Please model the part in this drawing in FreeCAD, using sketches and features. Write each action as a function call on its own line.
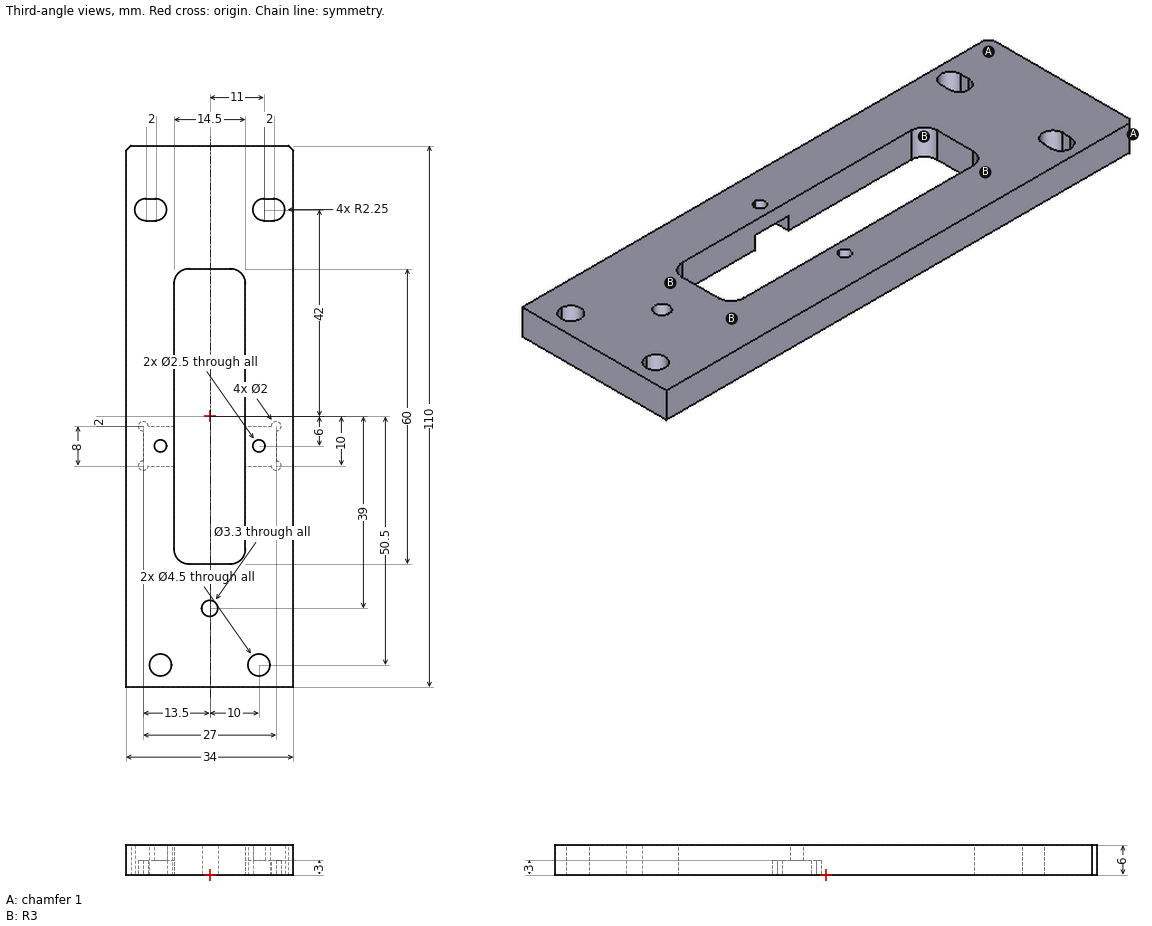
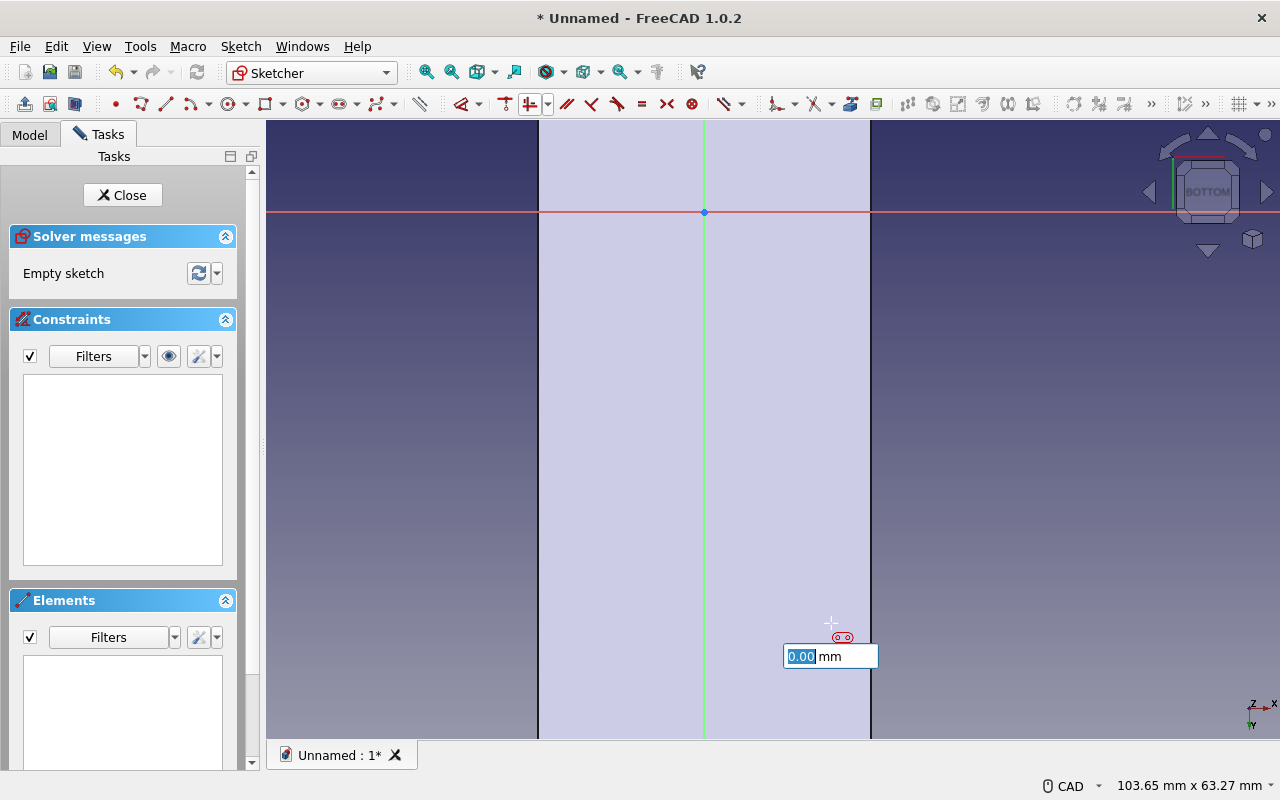
click(822, 645)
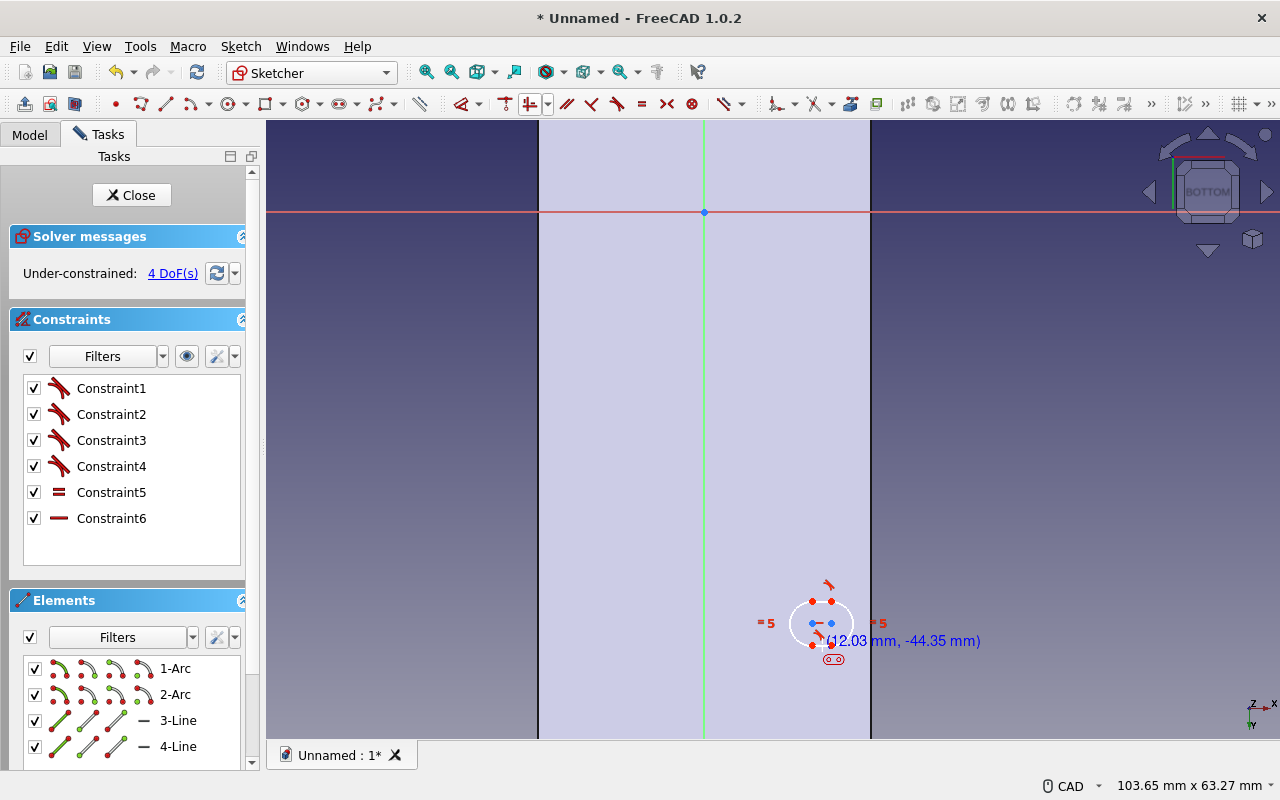
click(577, 623)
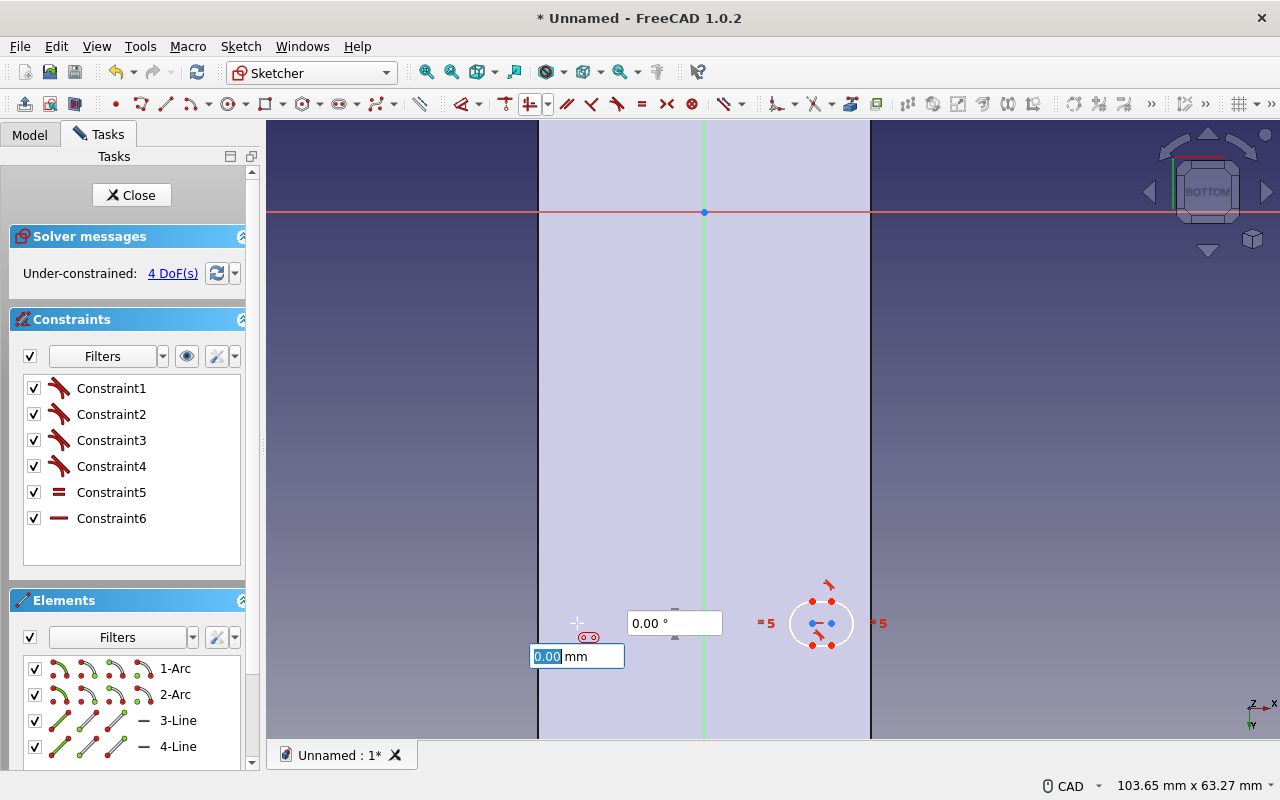
click(597, 623)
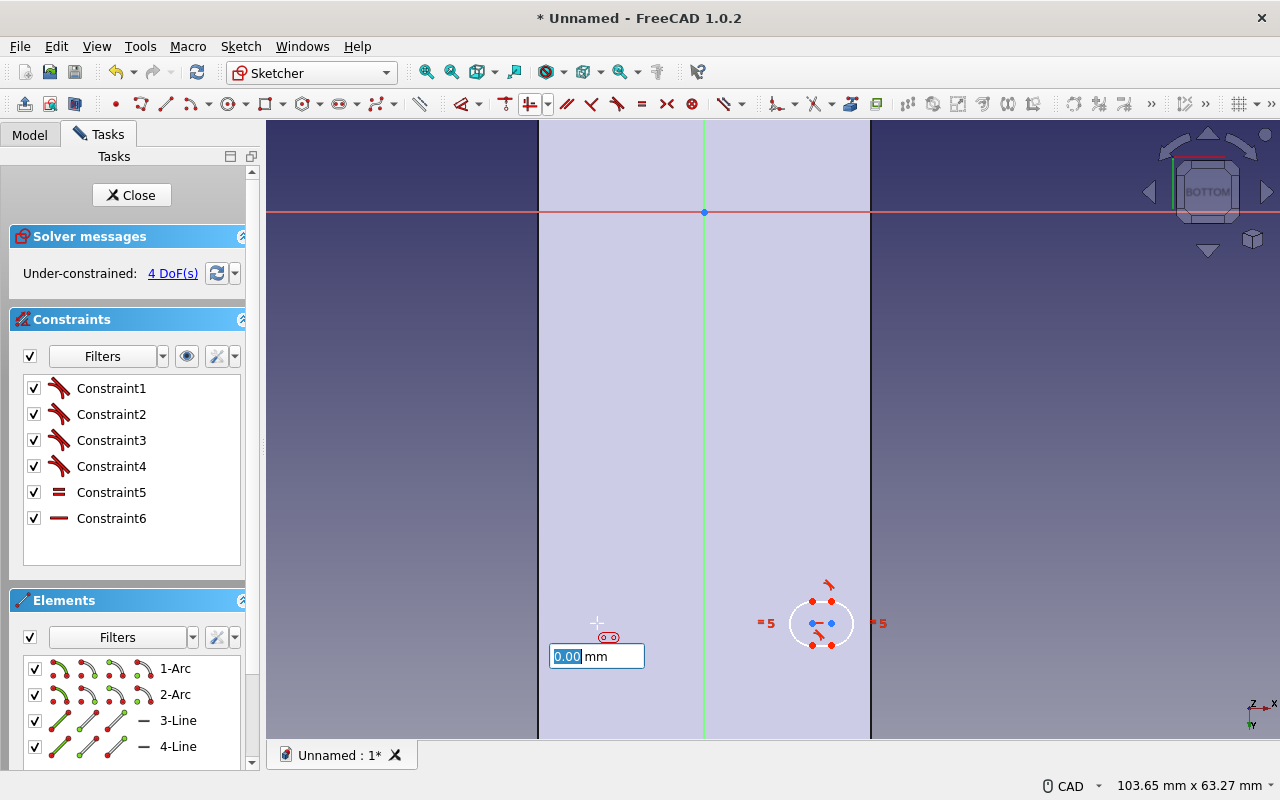
click(587, 645)
key(Escape)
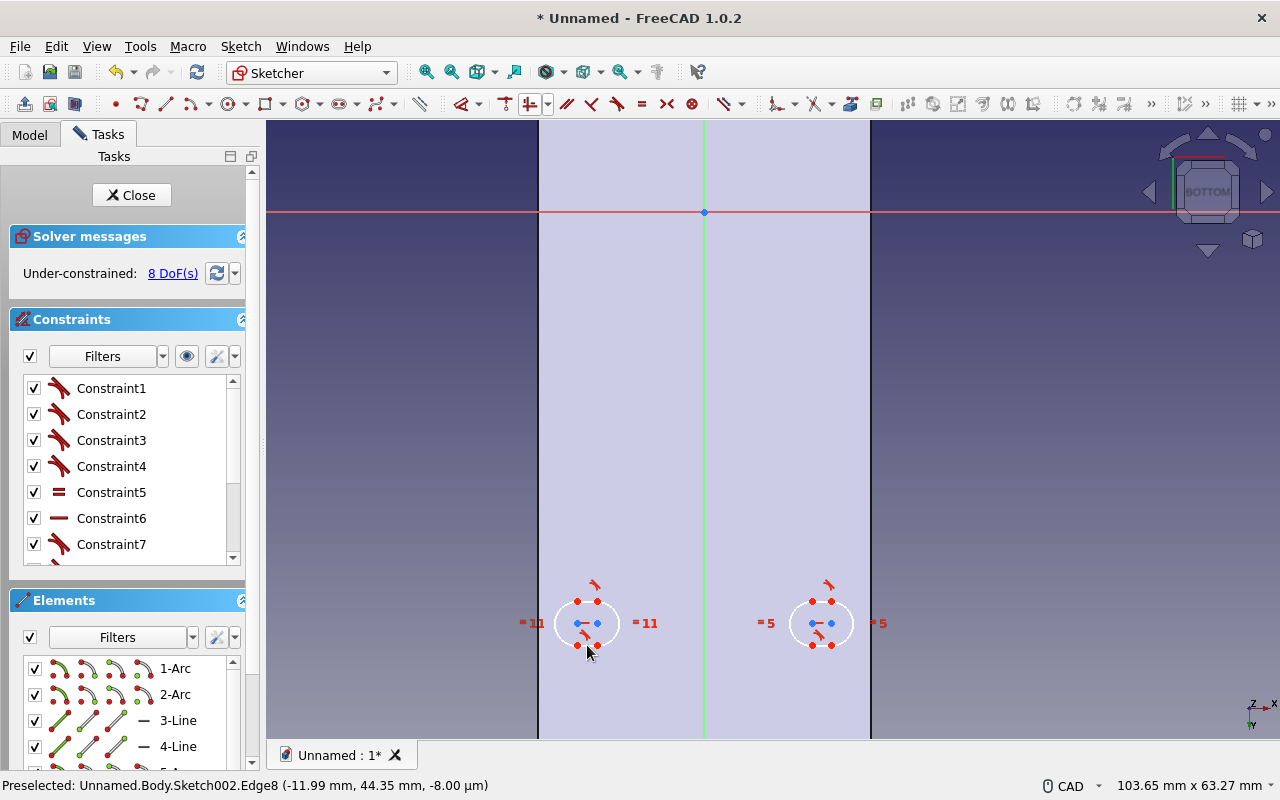
click(794, 611)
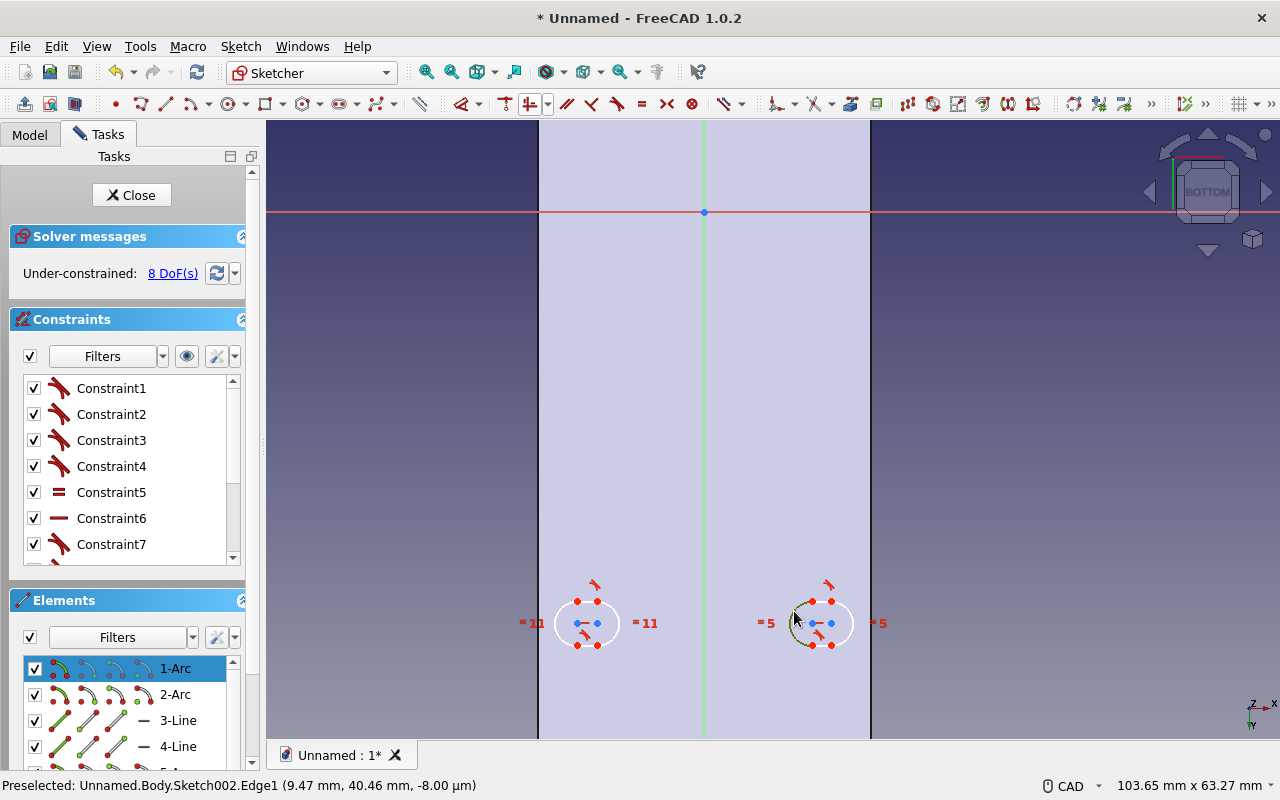
click(559, 611)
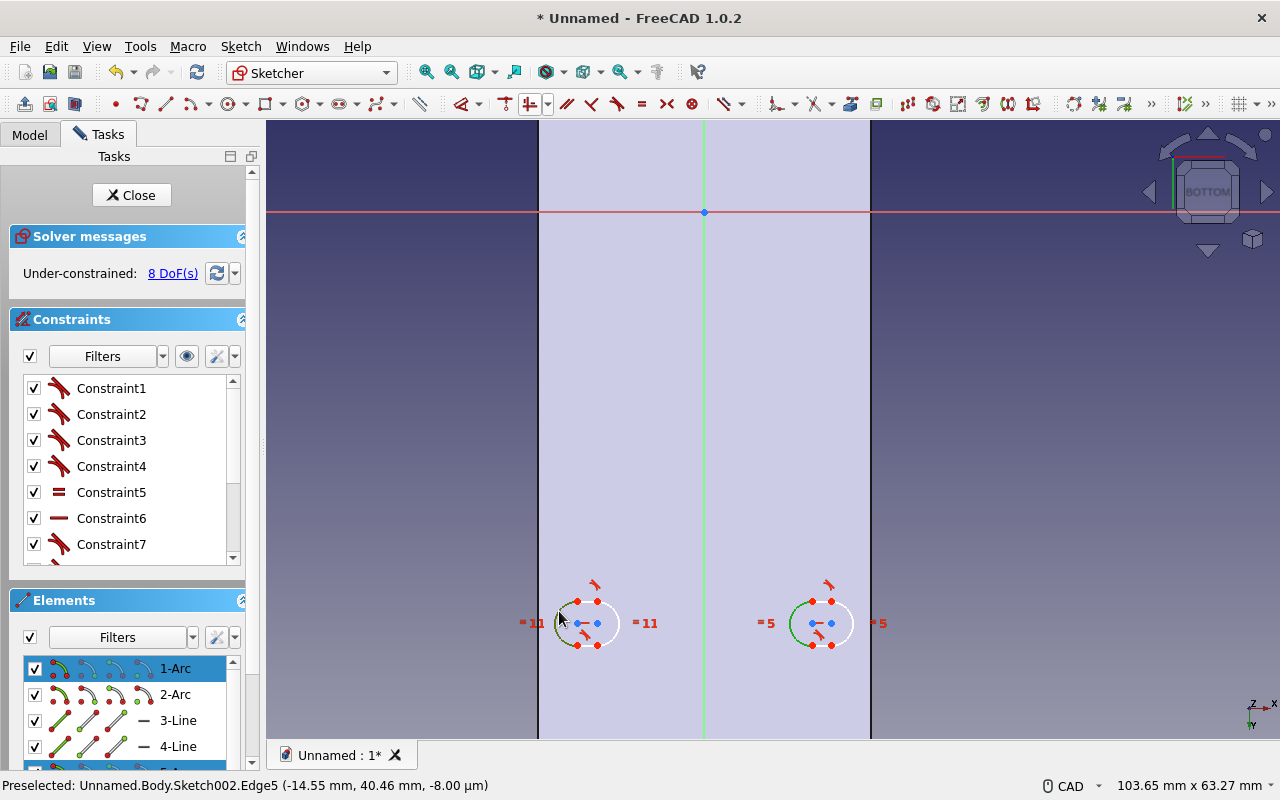
key(e)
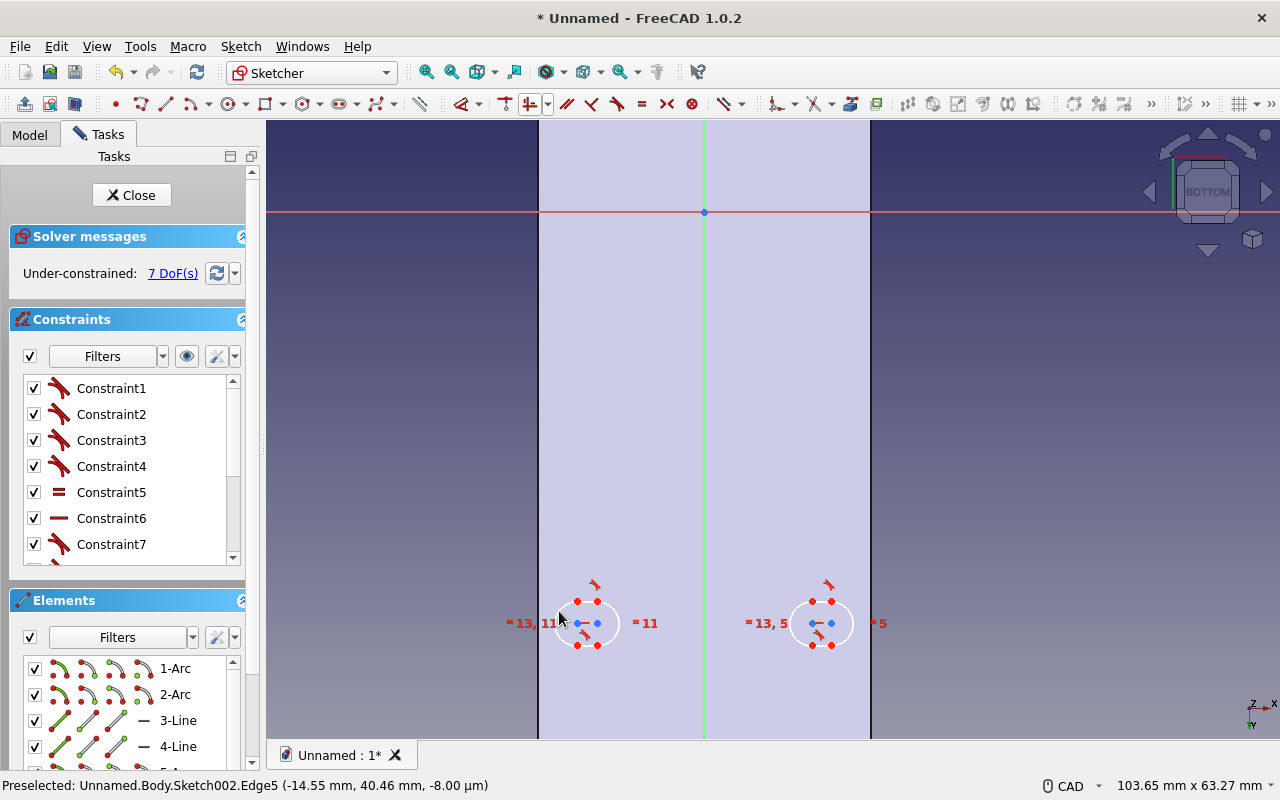
click(831, 624)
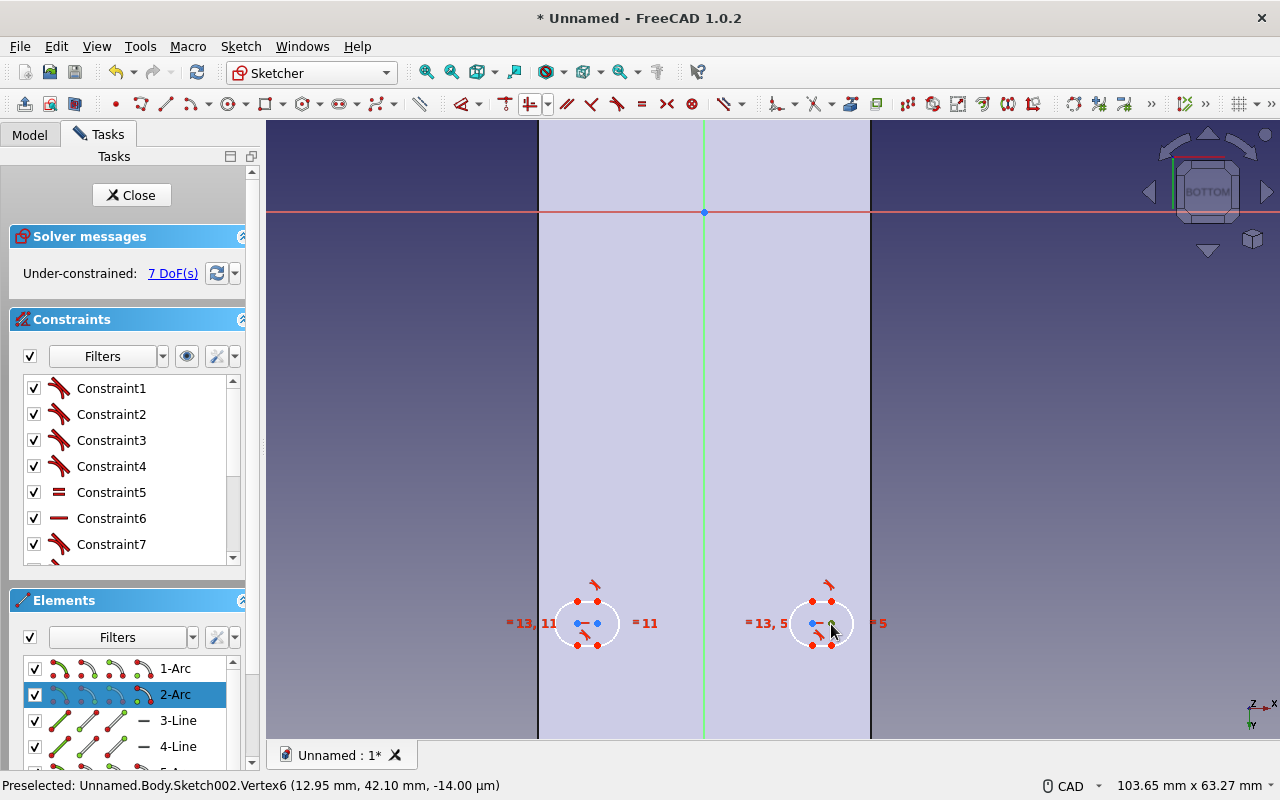
click(577, 624)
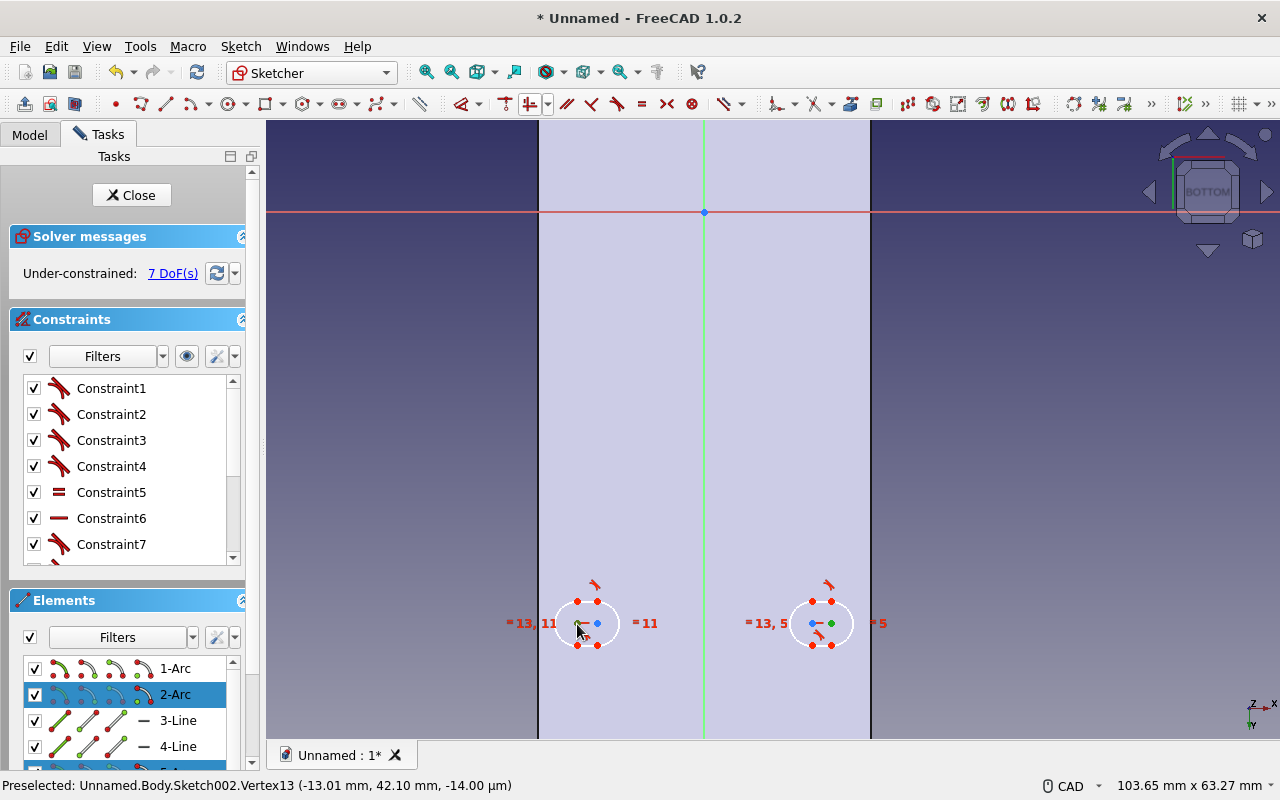
click(704, 671)